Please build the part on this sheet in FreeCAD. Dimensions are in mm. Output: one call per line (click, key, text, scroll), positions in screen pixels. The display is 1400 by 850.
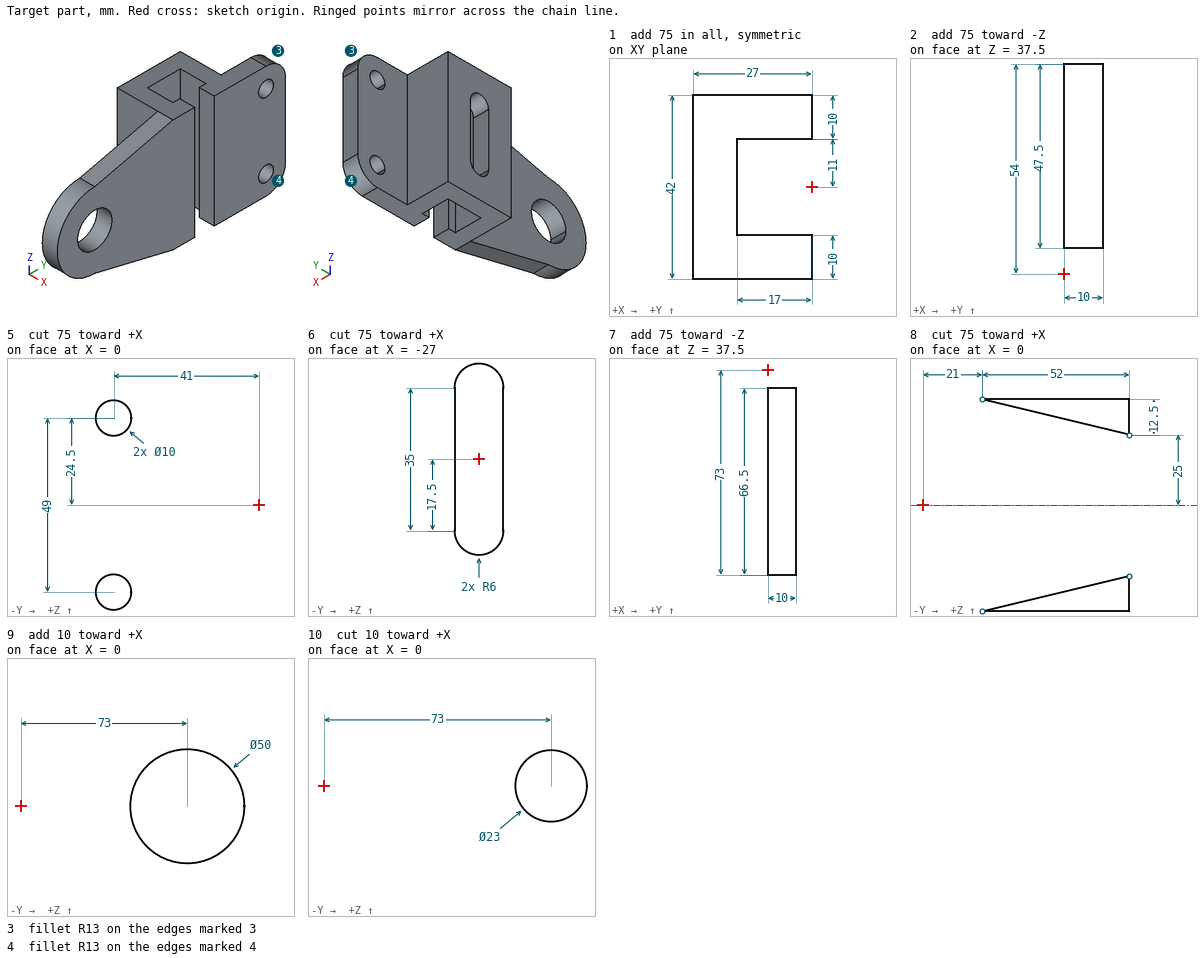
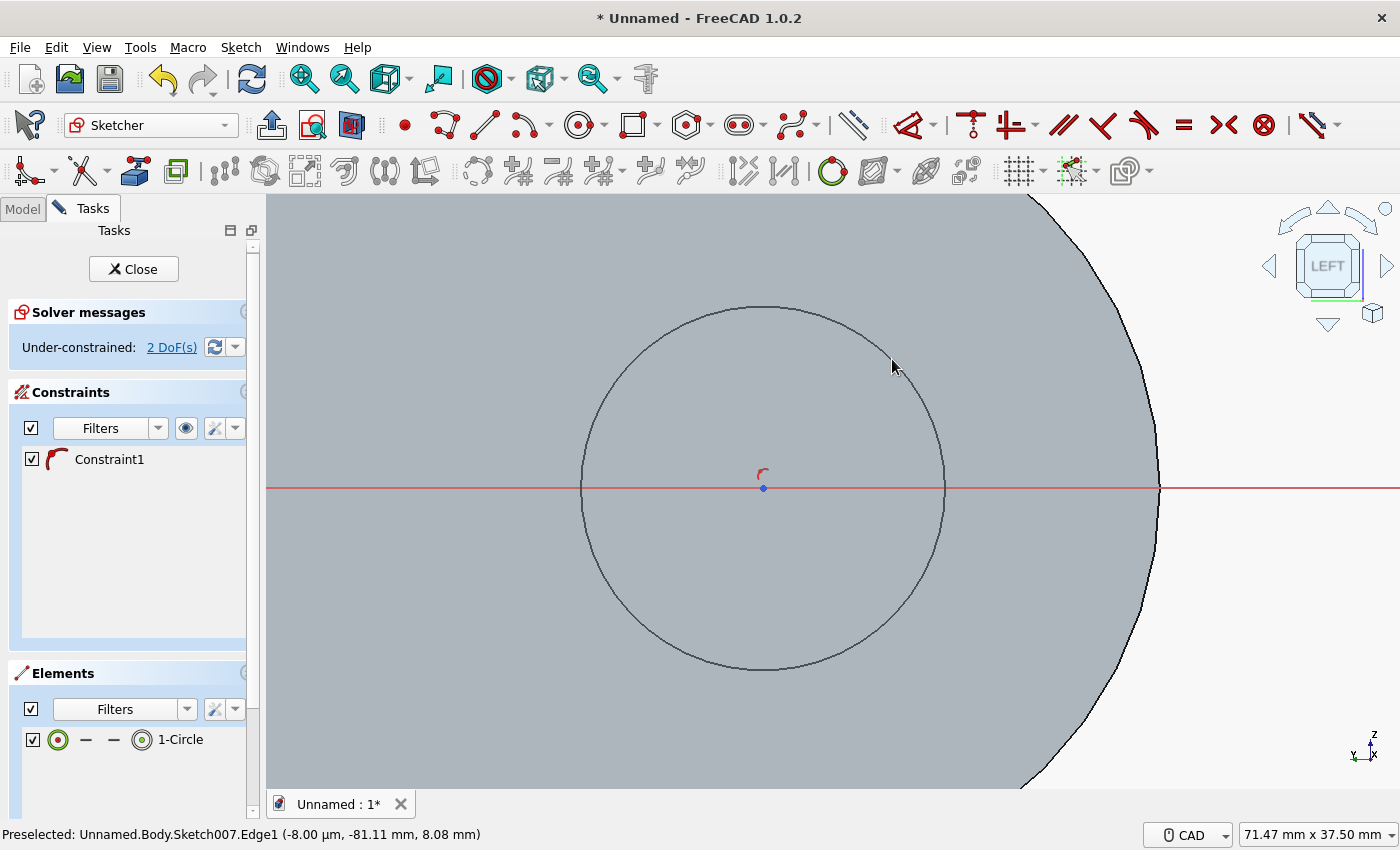
key(d)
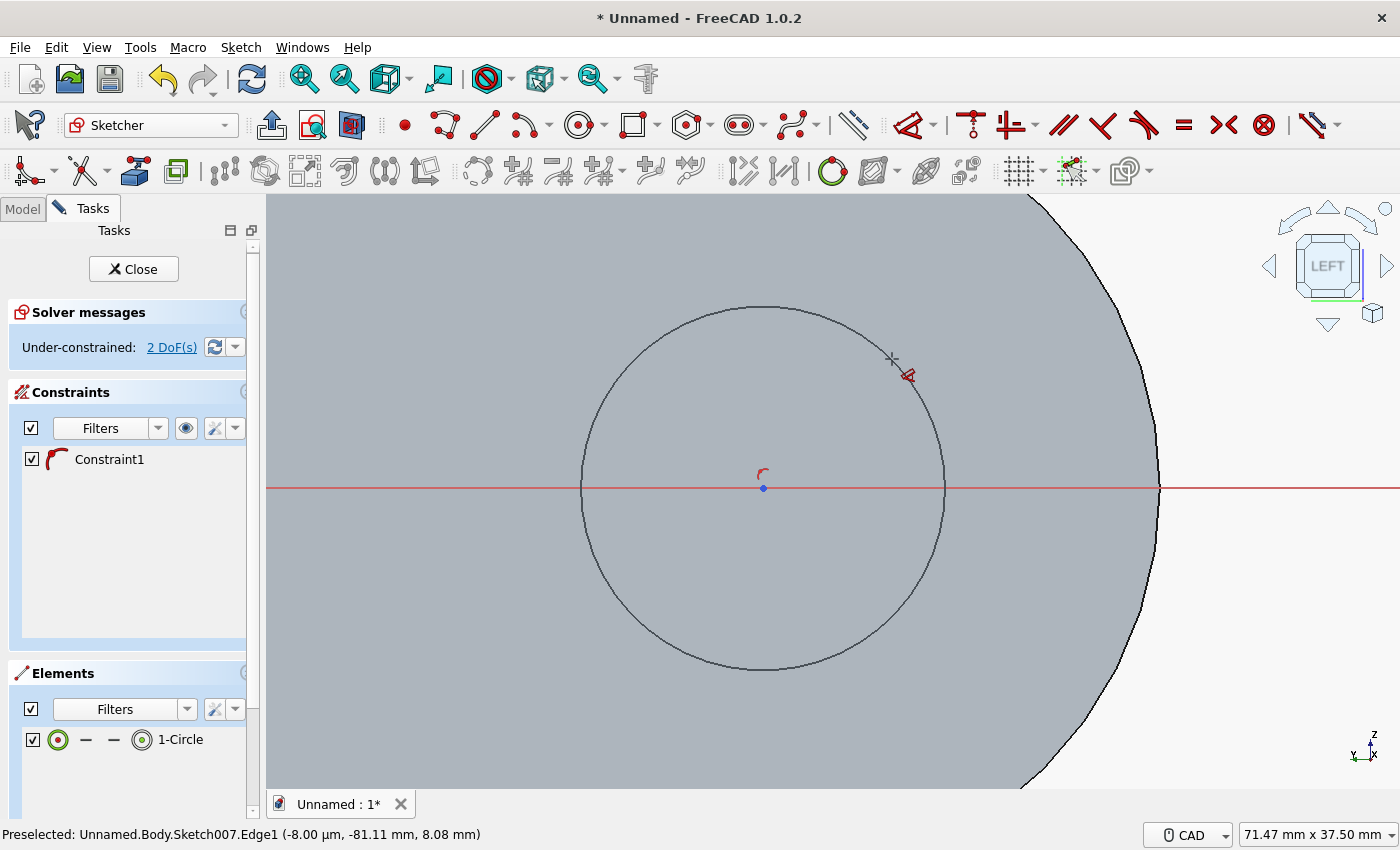
click(891, 359)
click(914, 336)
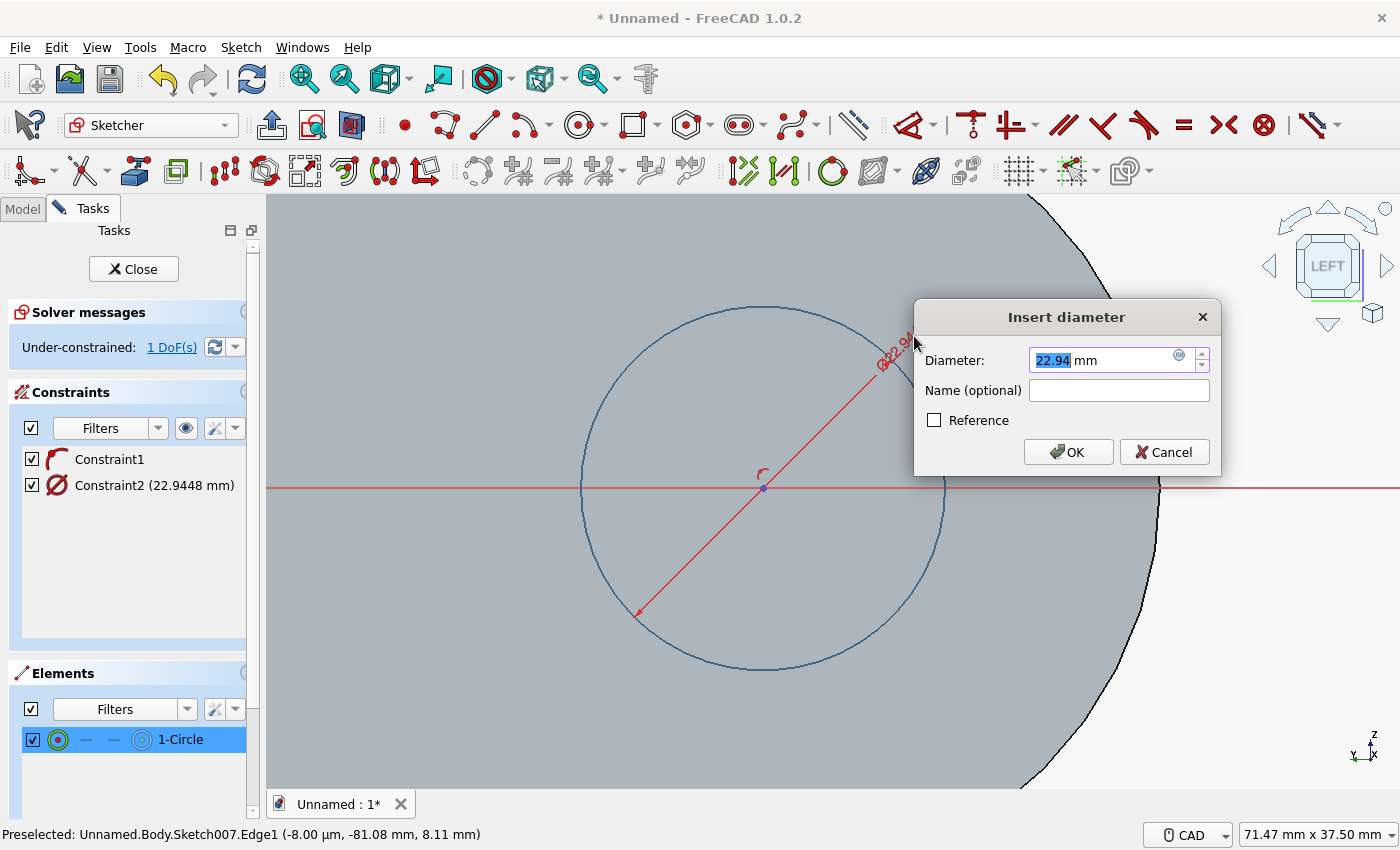
text(23)
key(Return)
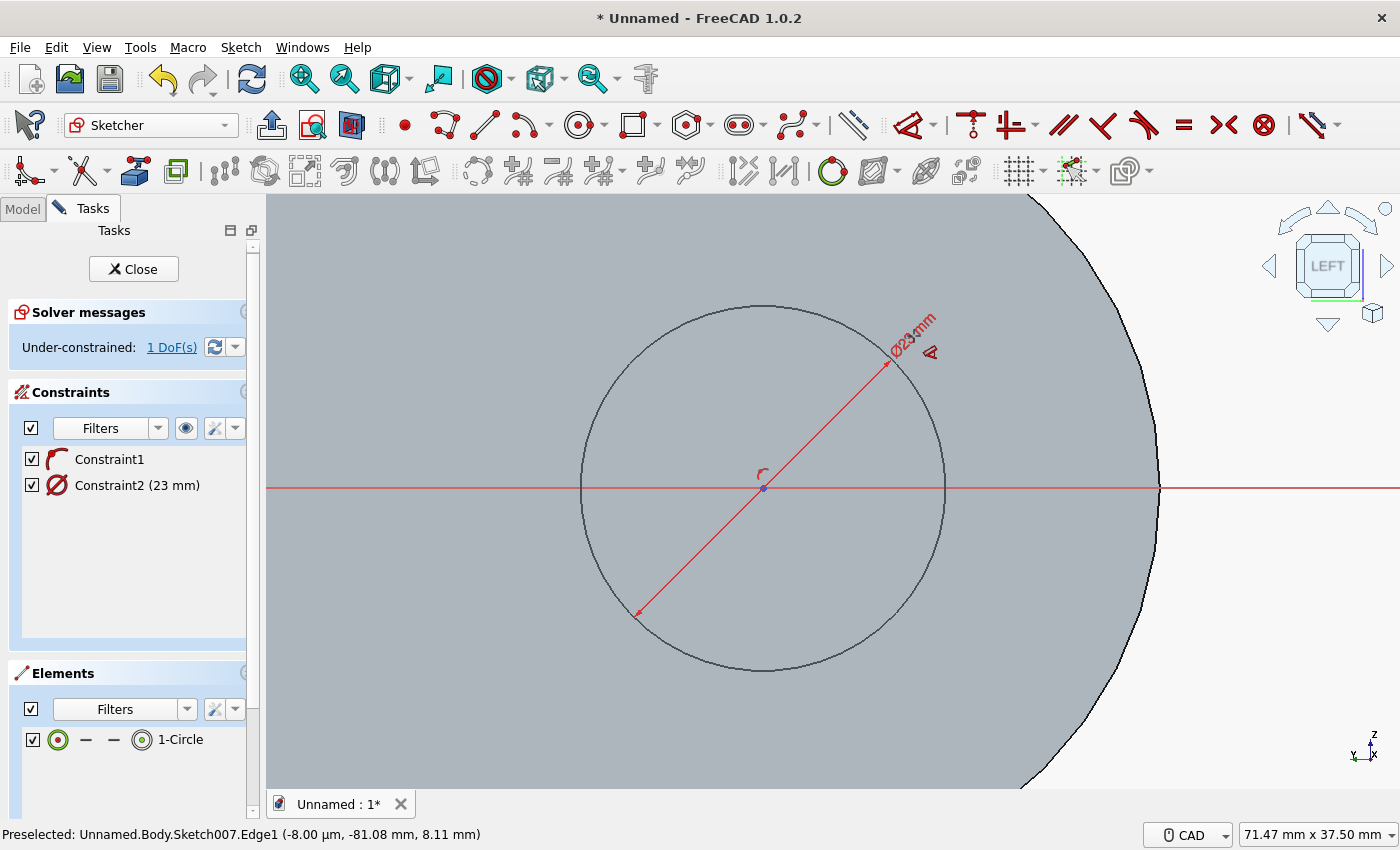
click(763, 488)
click(529, 522)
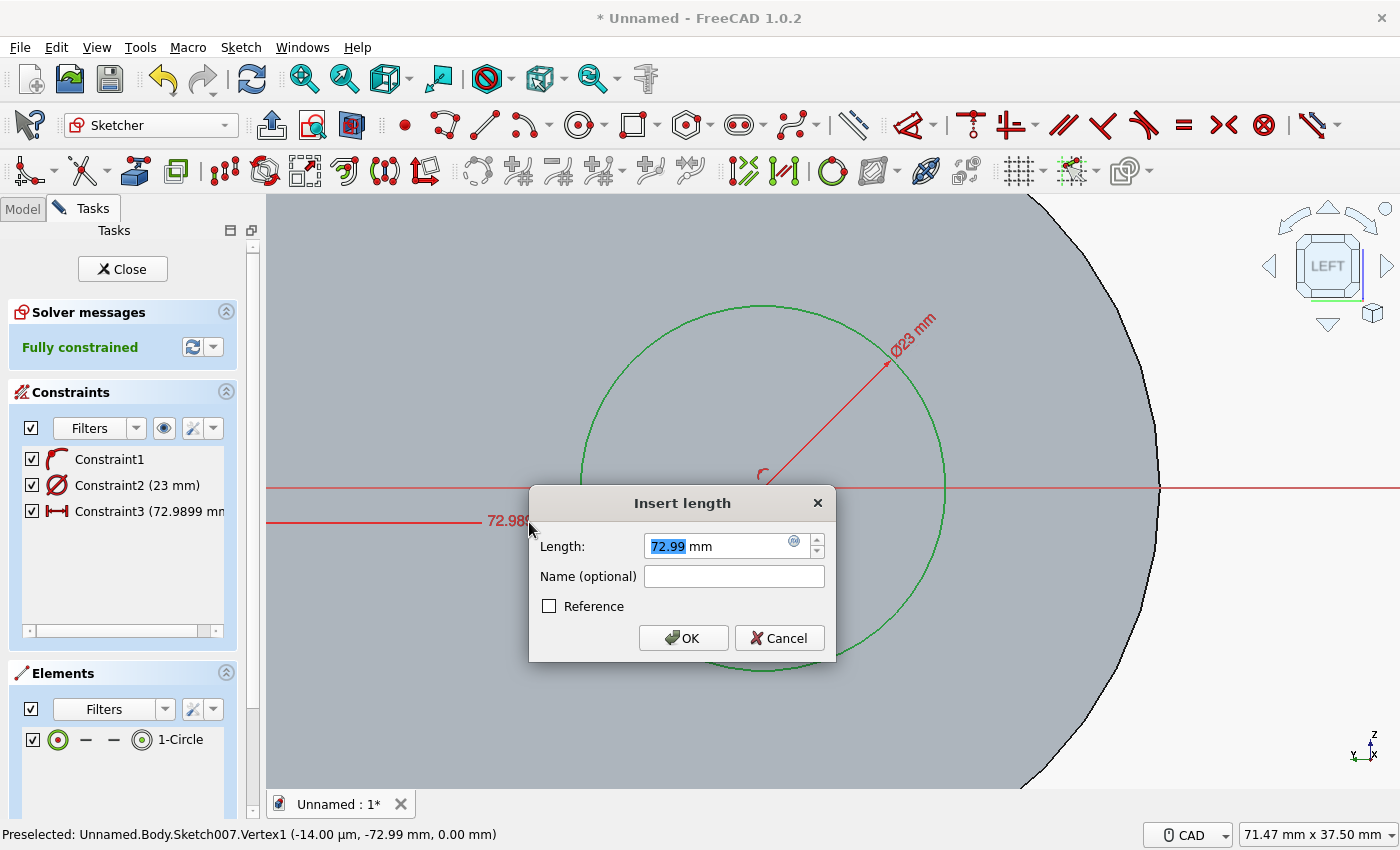
text(73)
key(Return)
key(Escape)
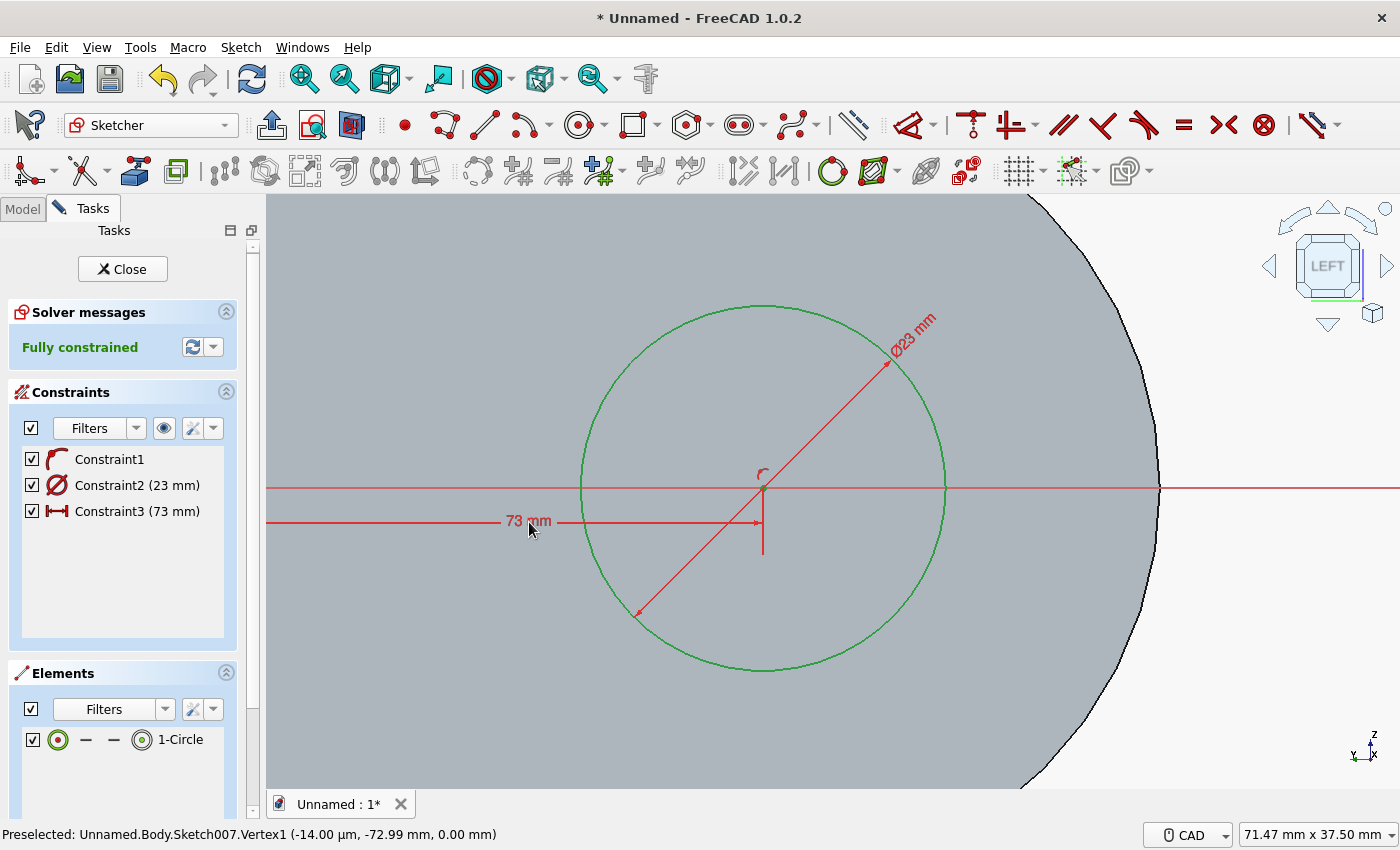
click(123, 269)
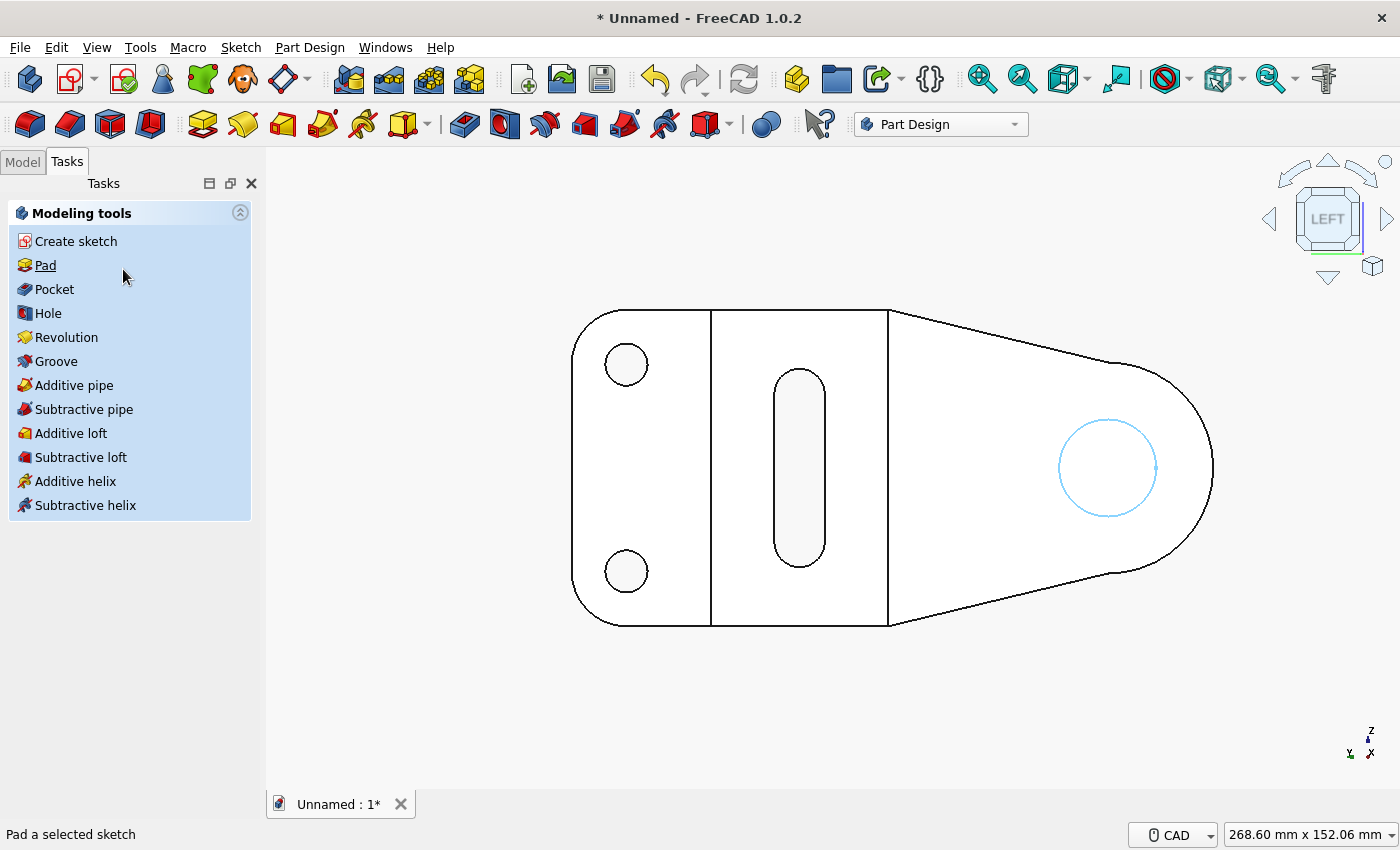
click(466, 124)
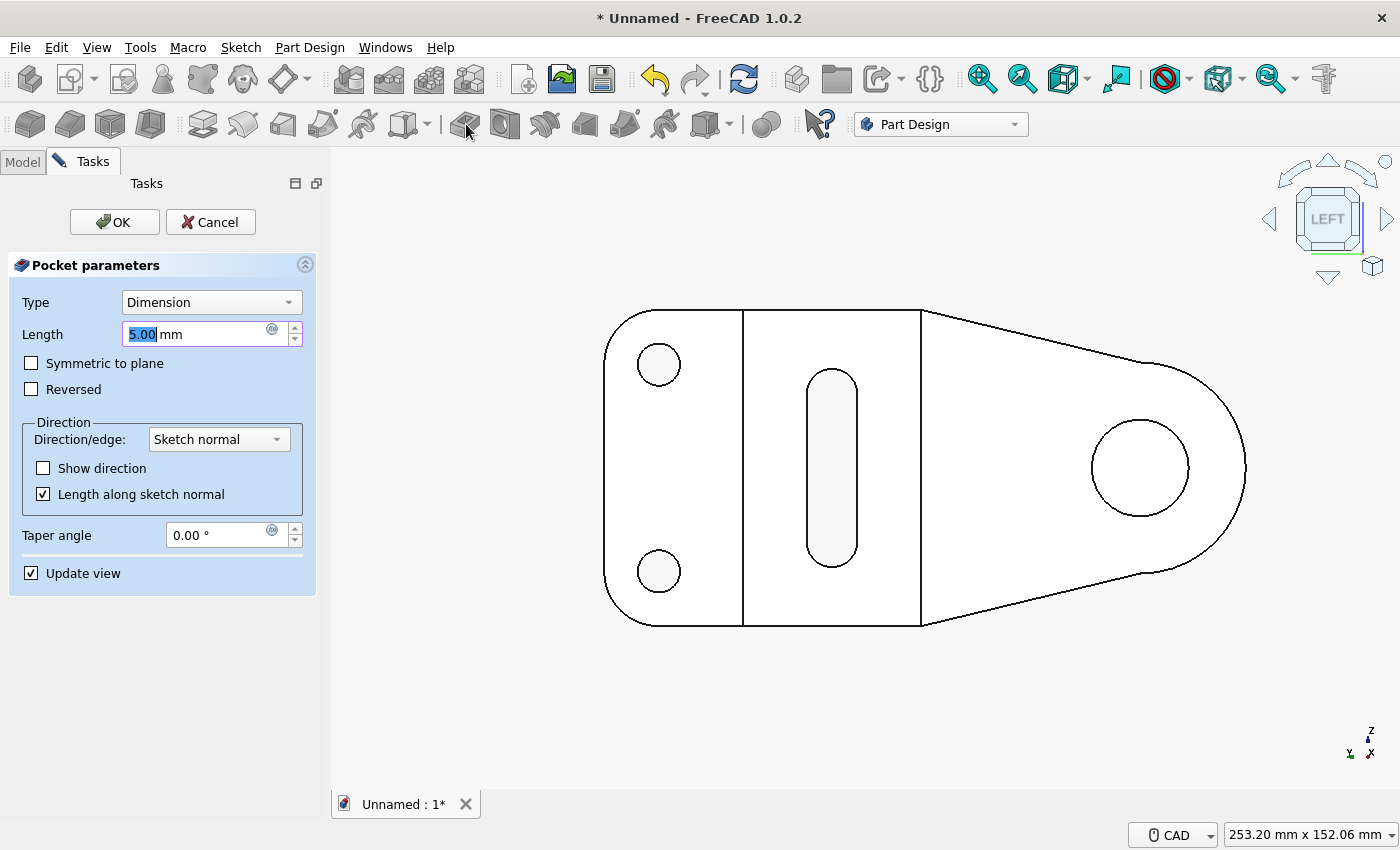
text(10)
key(Tab)